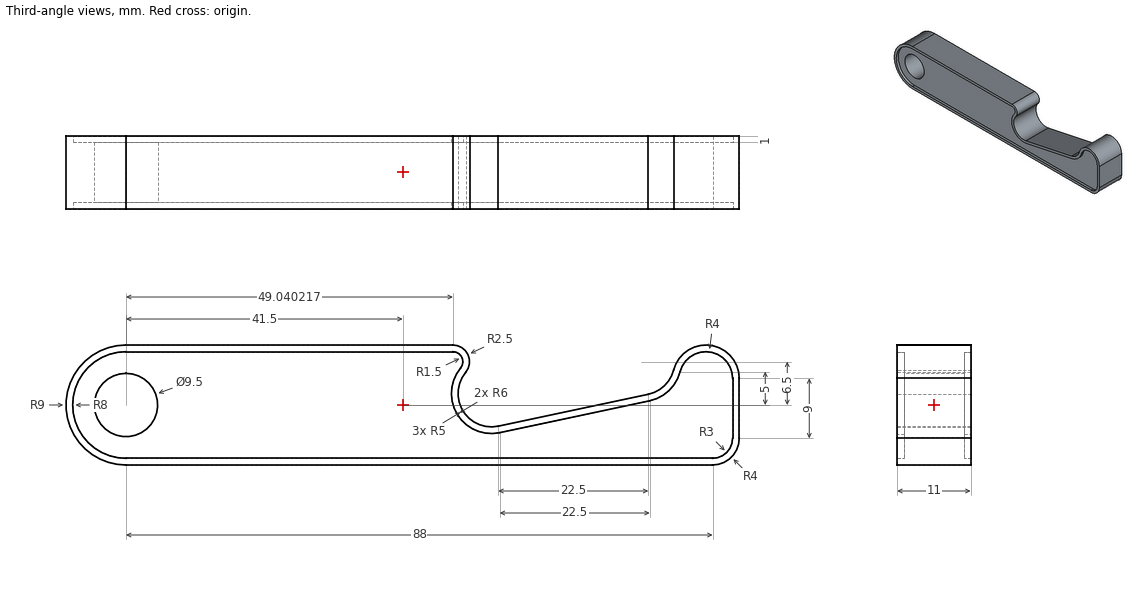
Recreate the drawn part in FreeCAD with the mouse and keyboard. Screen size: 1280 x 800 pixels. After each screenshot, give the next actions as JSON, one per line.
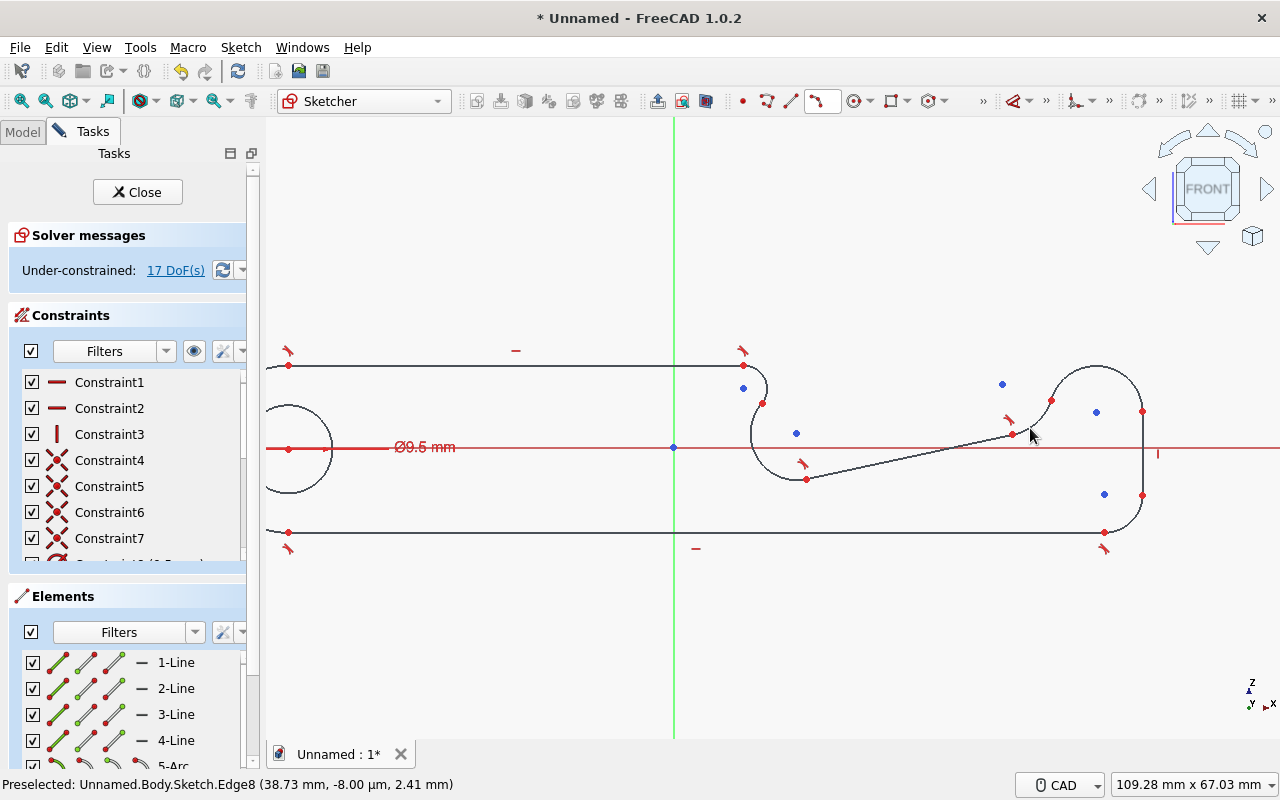
{"action": "scroll", "coordinate": [767, 388], "scroll_direction": "down", "scroll_amount": 2}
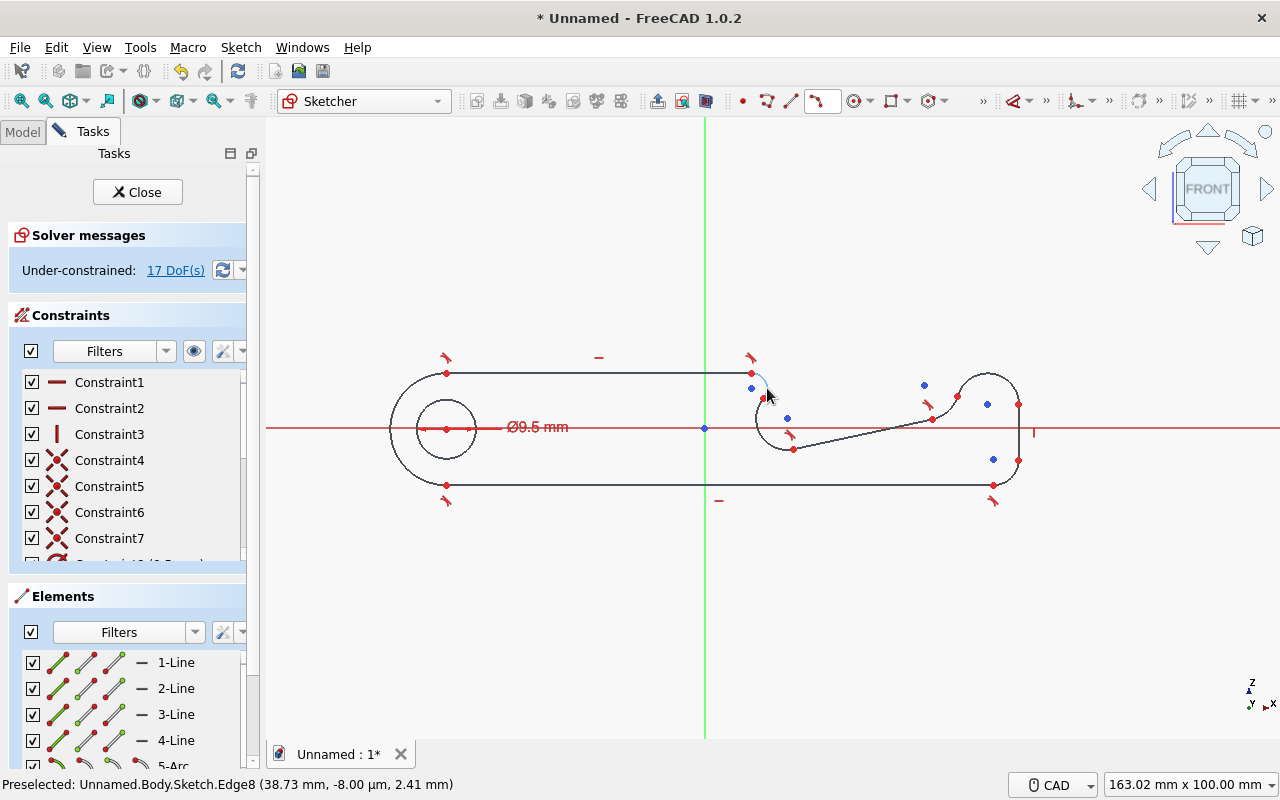
{"action": "scroll", "coordinate": [1019, 421], "scroll_direction": "up", "scroll_amount": 4}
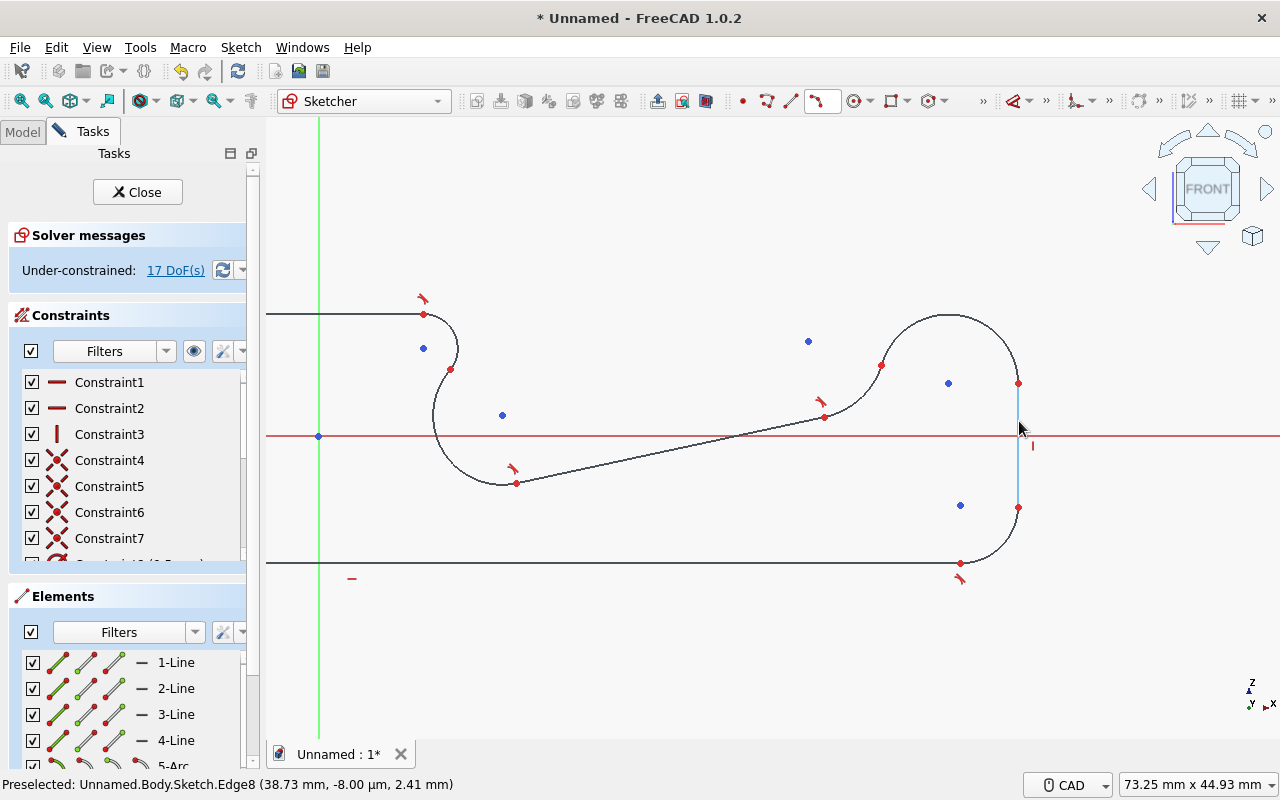
{"action": "left_click", "coordinate": [1018, 420]}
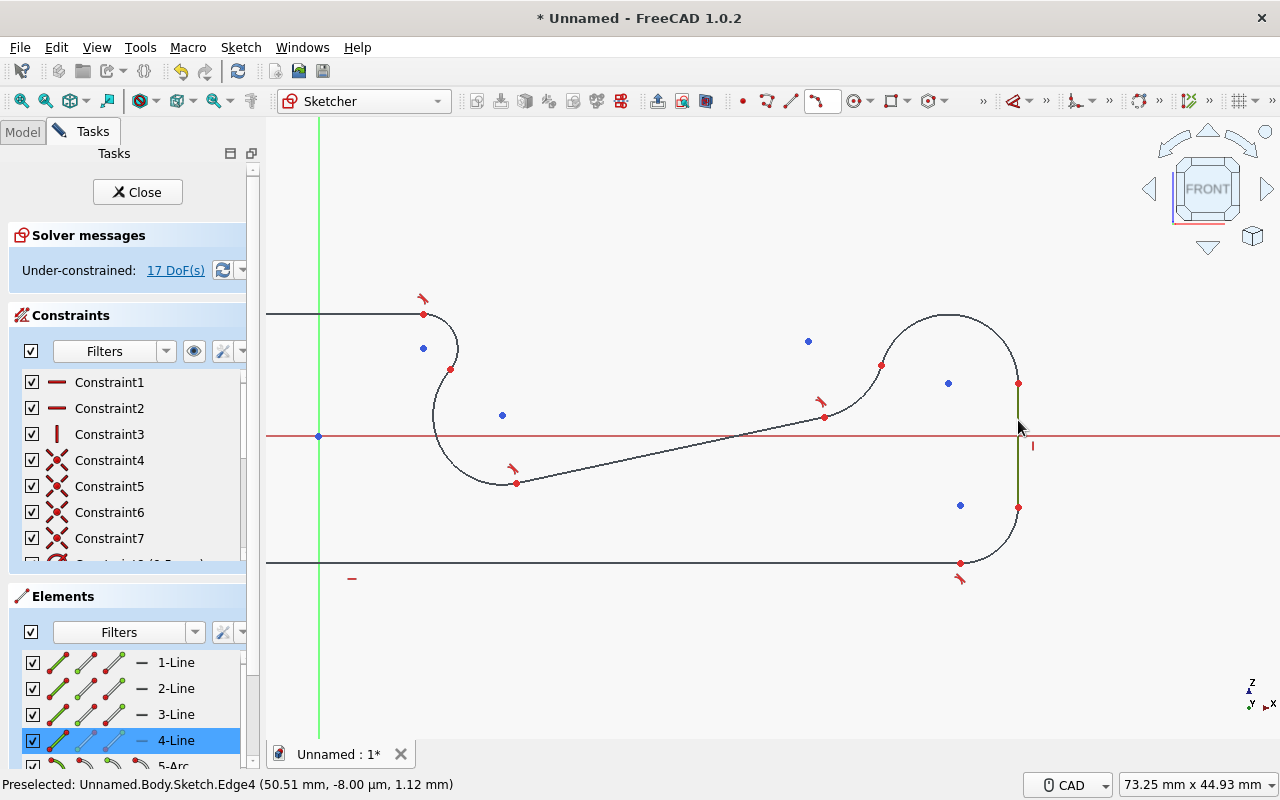
{"action": "left_click", "coordinate": [993, 331]}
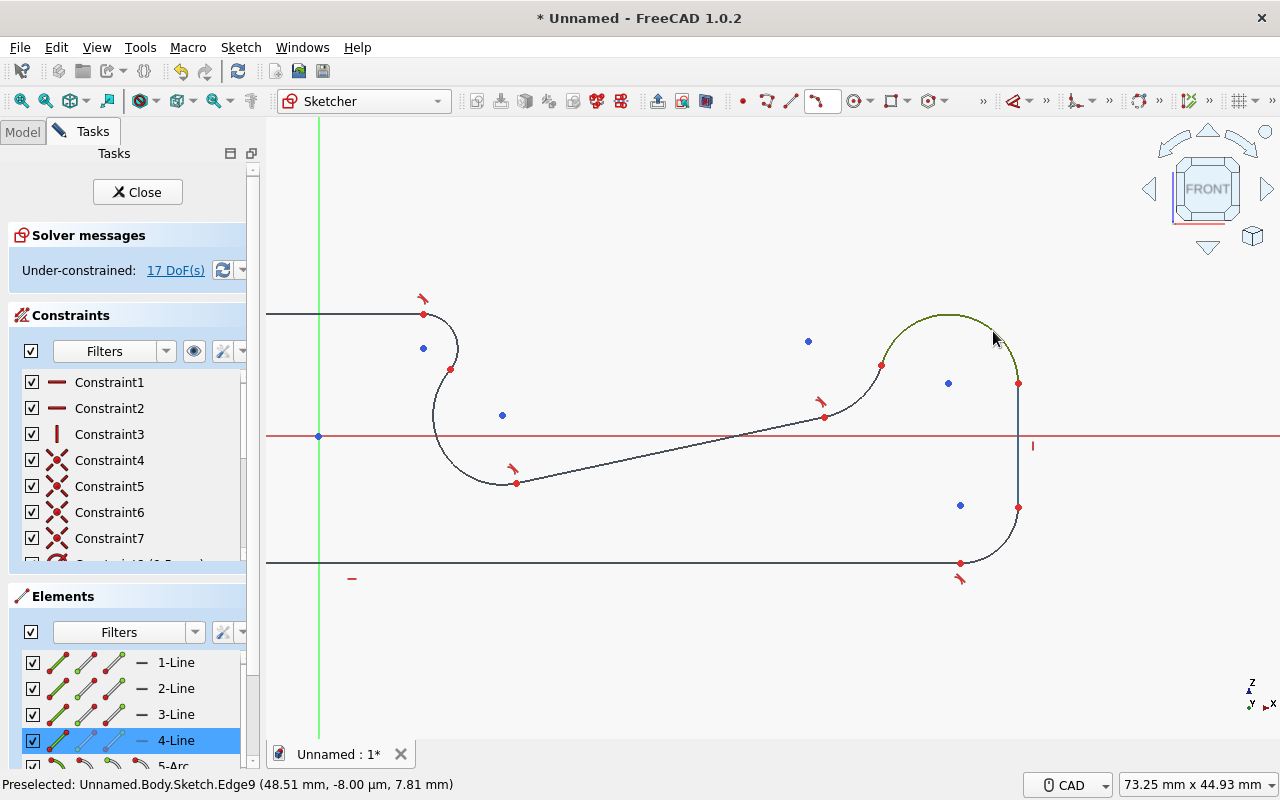
{"action": "key", "text": "t"}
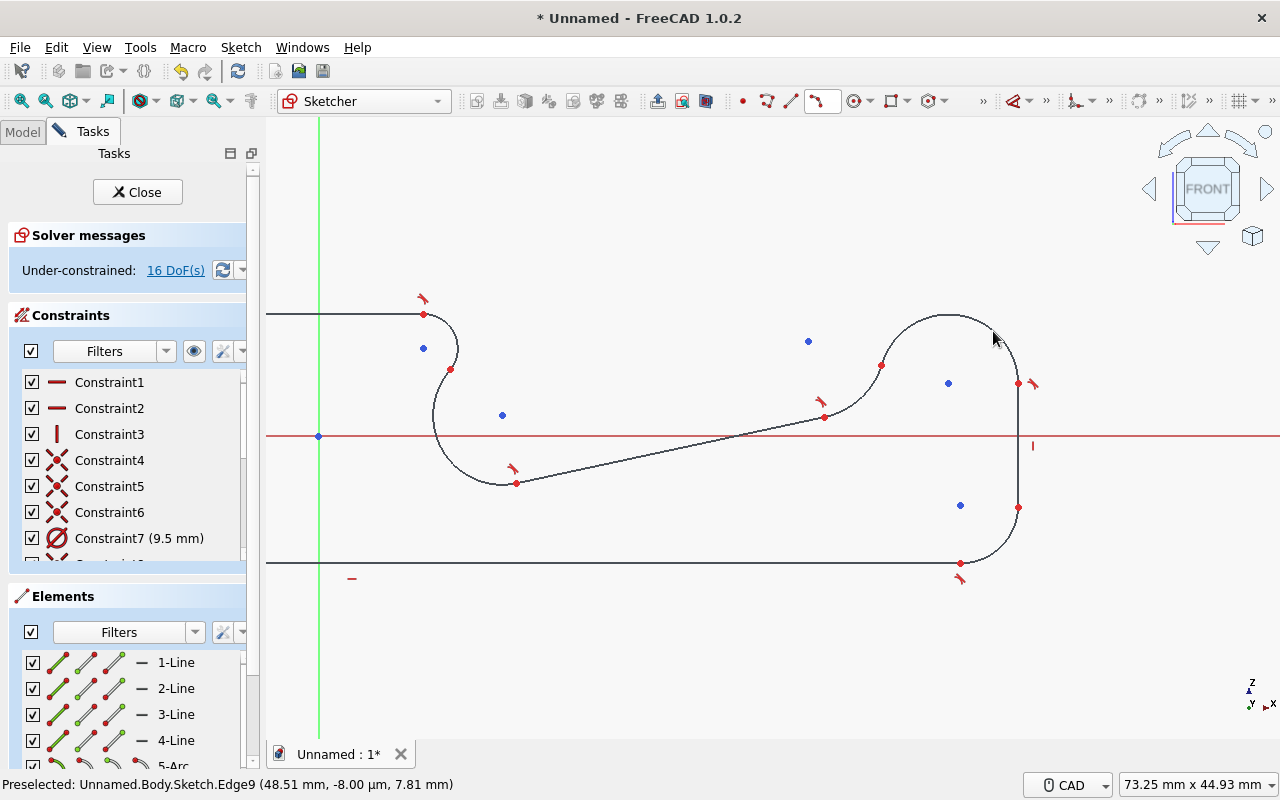
{"action": "left_click", "coordinate": [1018, 421]}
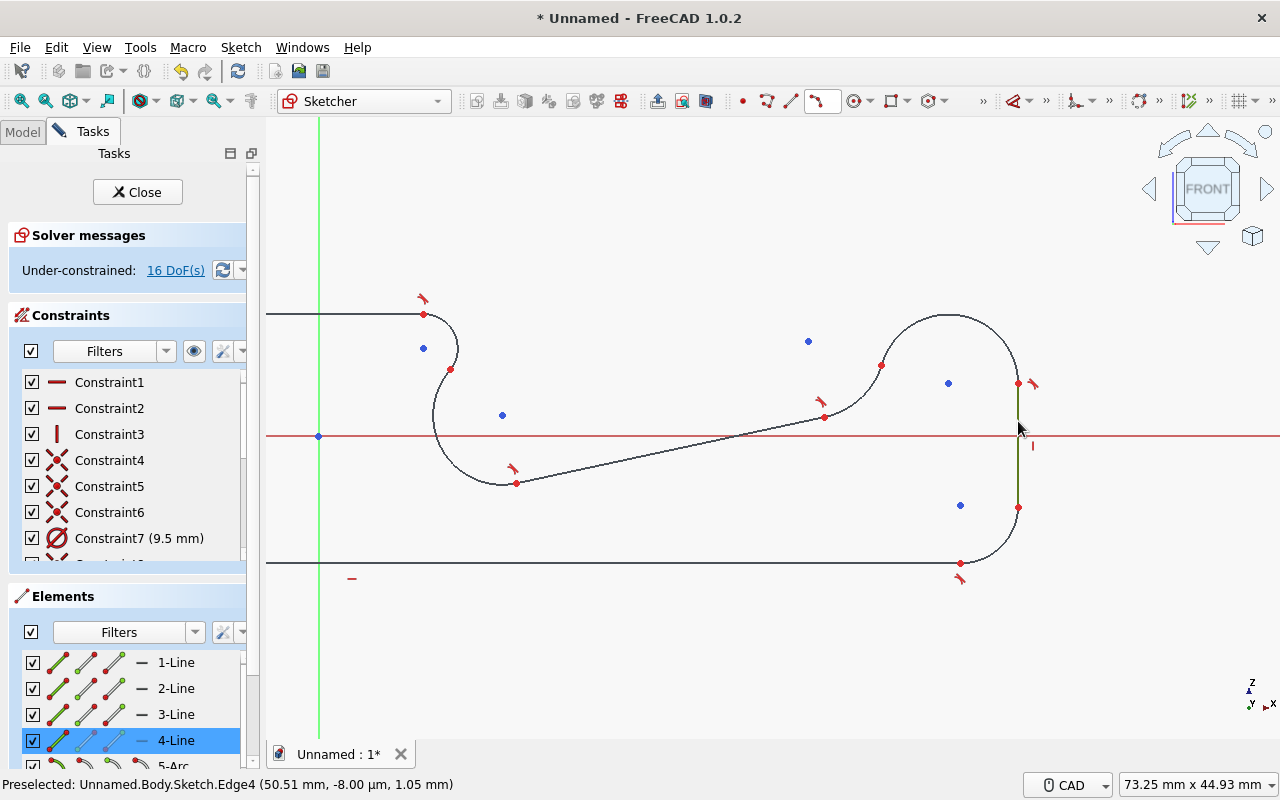
{"action": "left_click", "coordinate": [986, 557]}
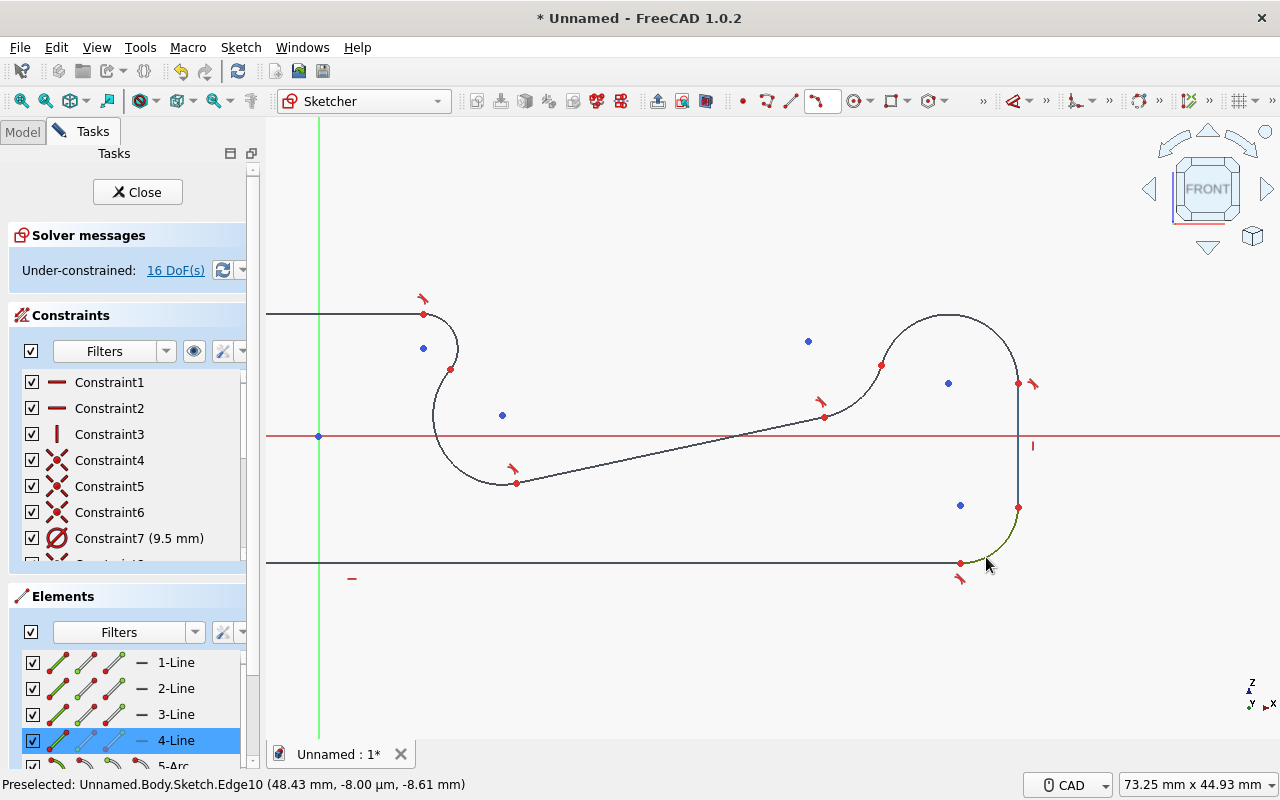
{"action": "key", "text": "t"}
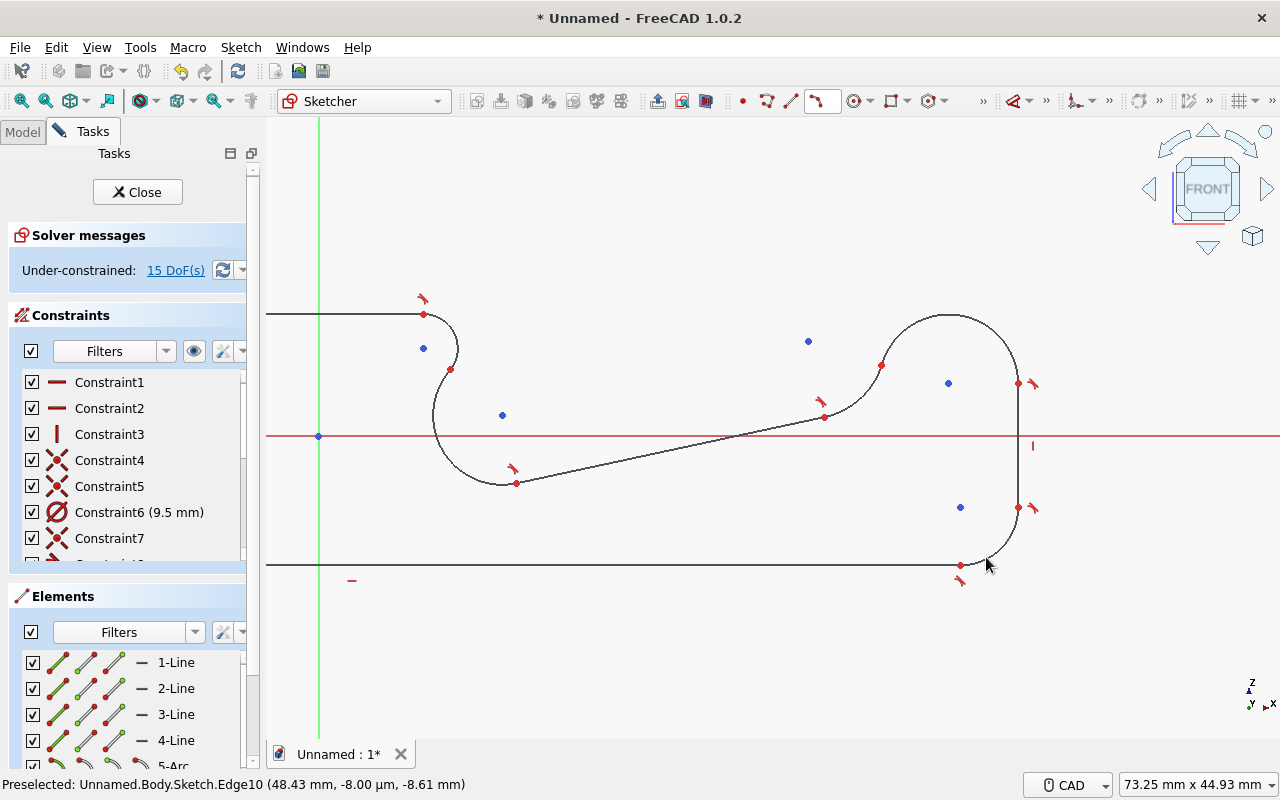
{"action": "left_click", "coordinate": [458, 348]}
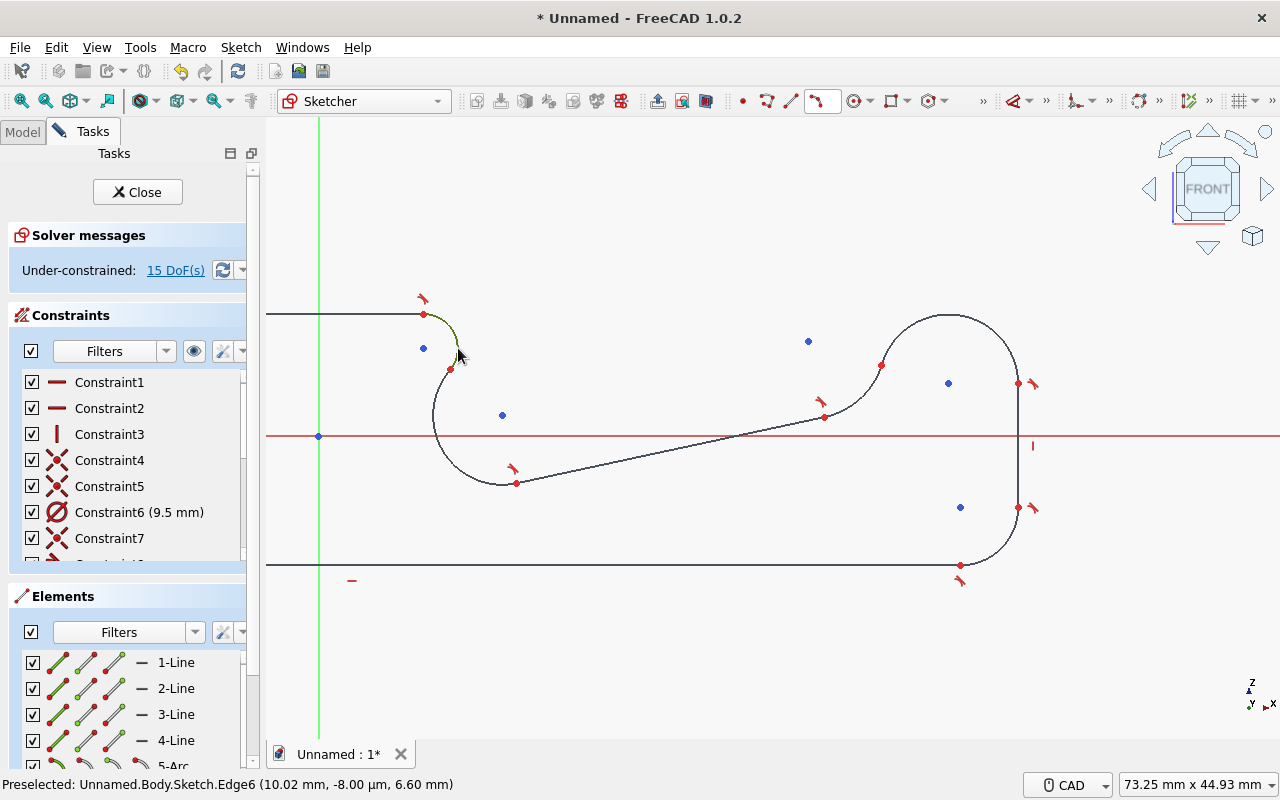
{"action": "left_click", "coordinate": [433, 417]}